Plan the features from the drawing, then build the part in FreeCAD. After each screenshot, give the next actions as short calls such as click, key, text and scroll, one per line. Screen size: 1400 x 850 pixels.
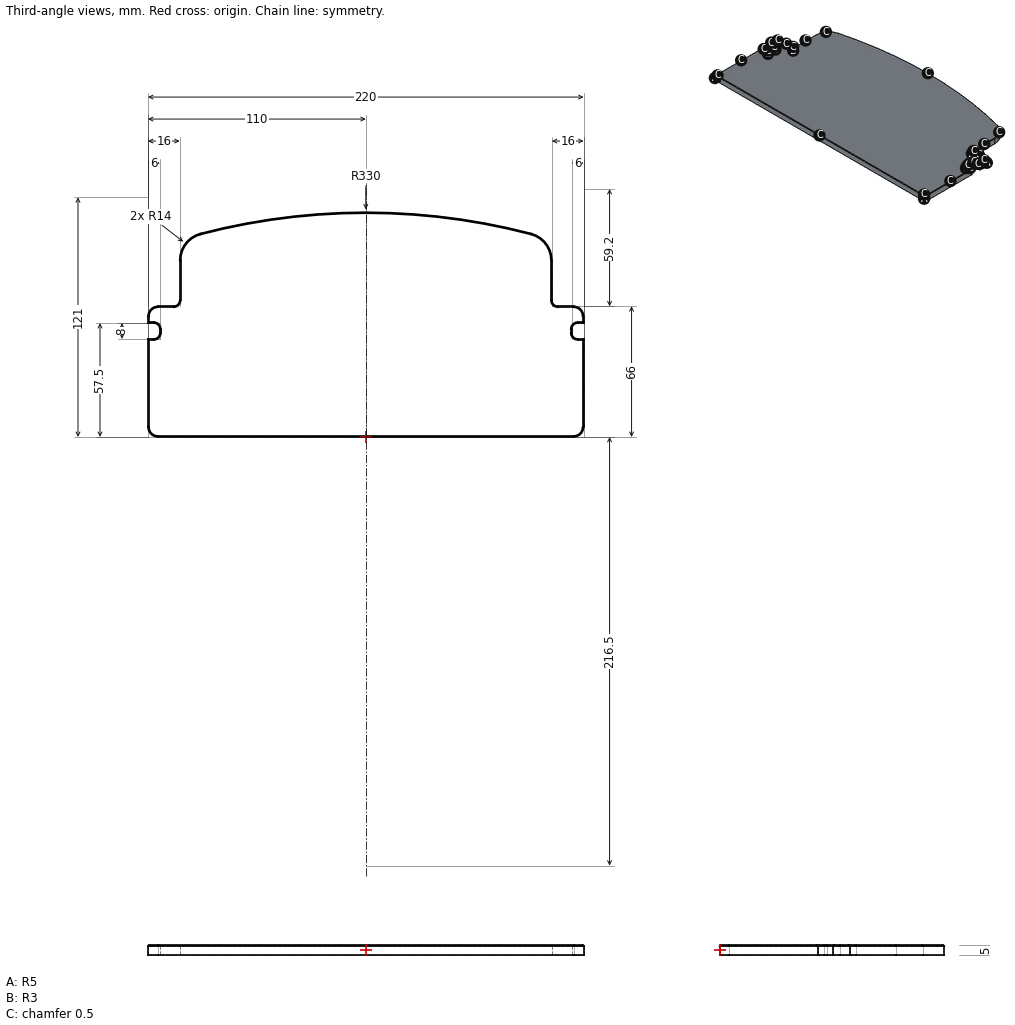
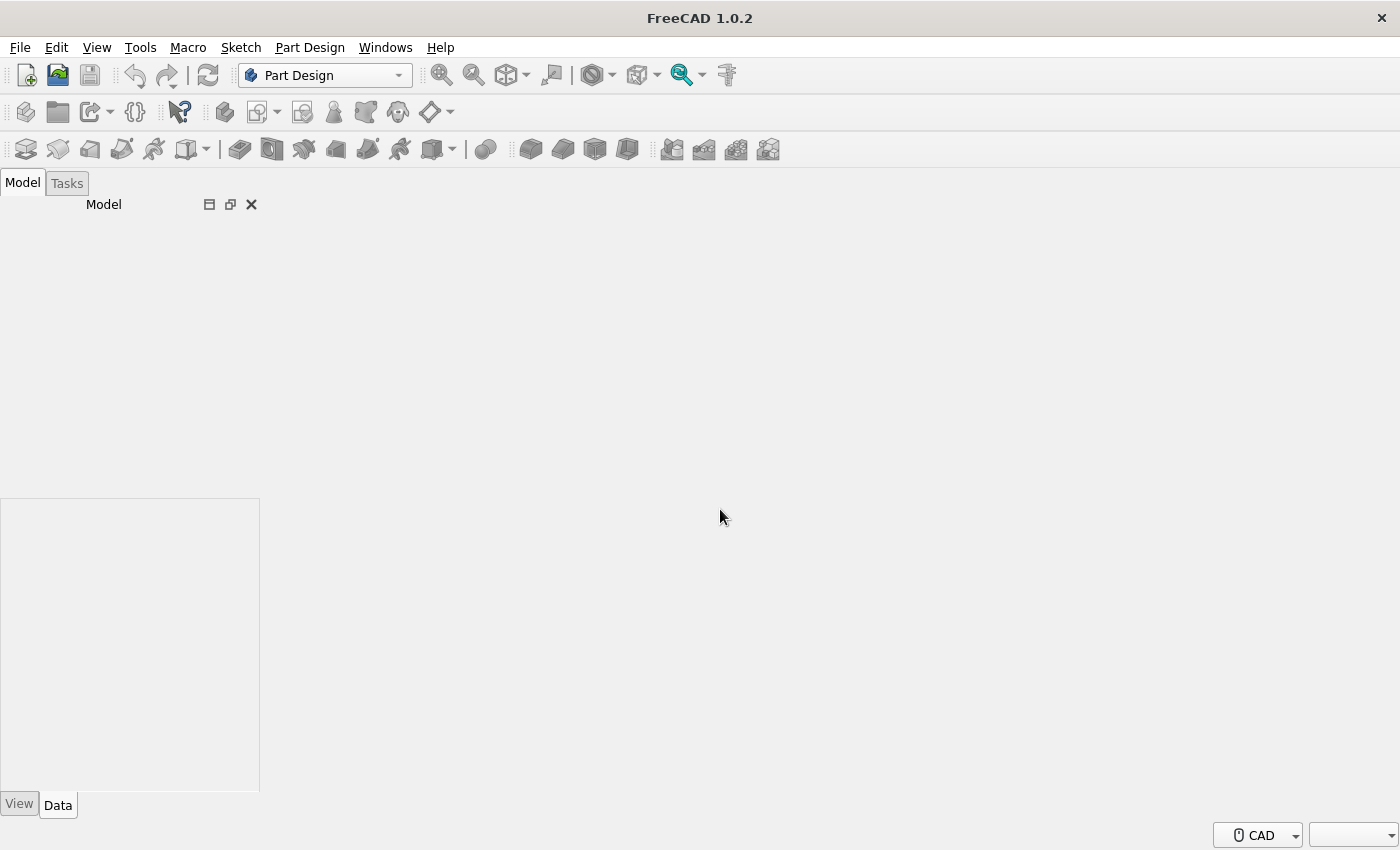
key(ctrl+n)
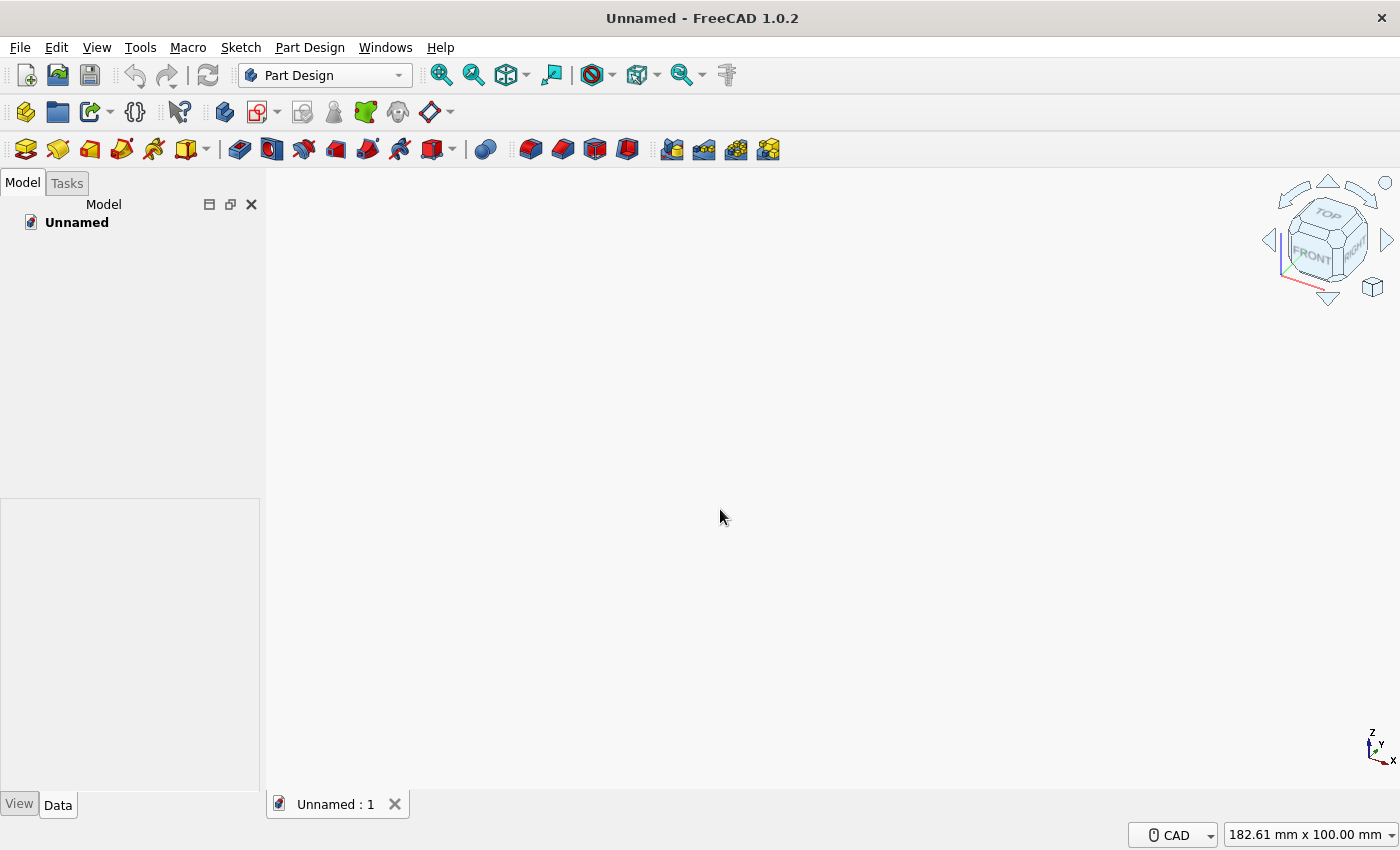
click(258, 112)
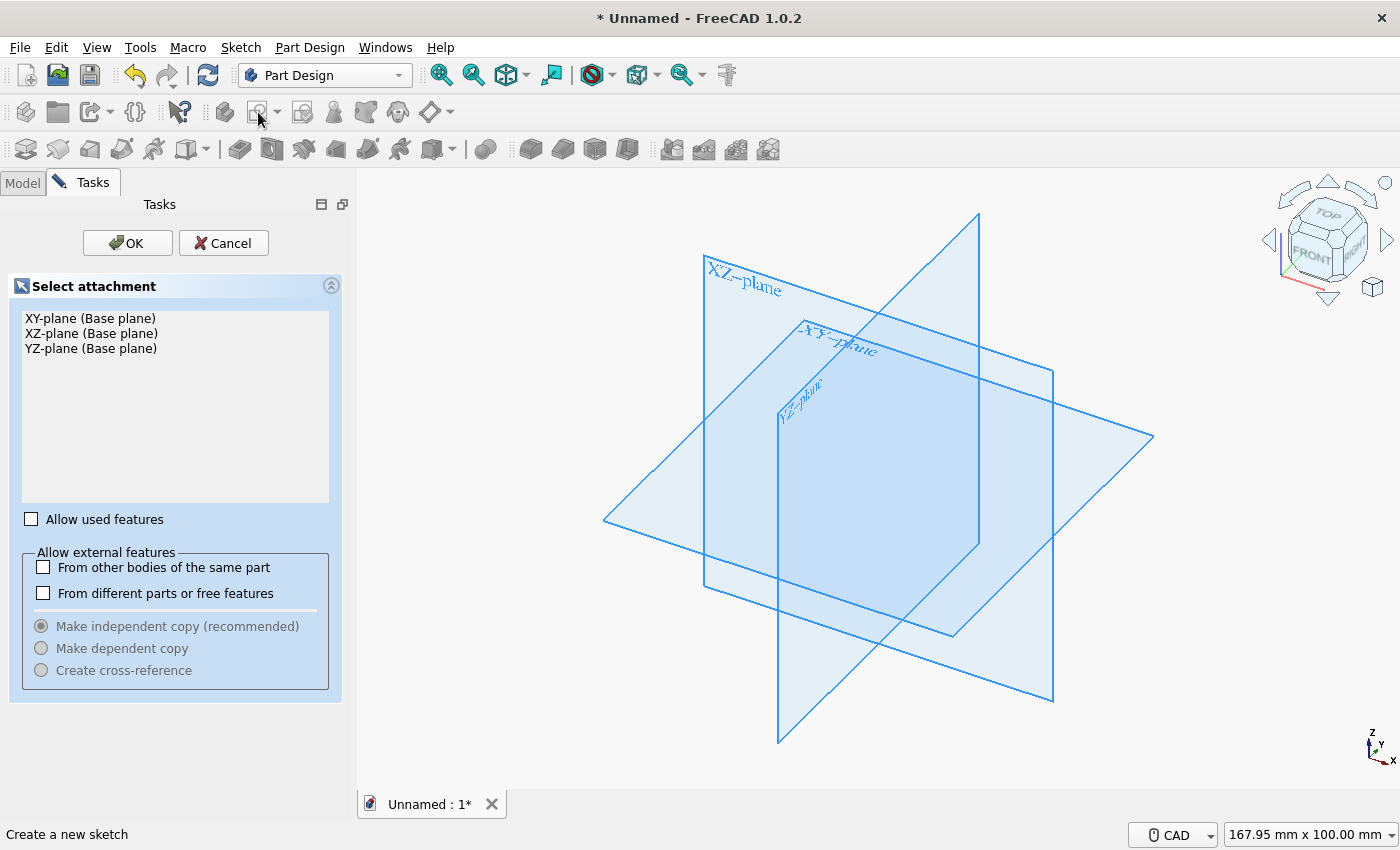
click(82, 318)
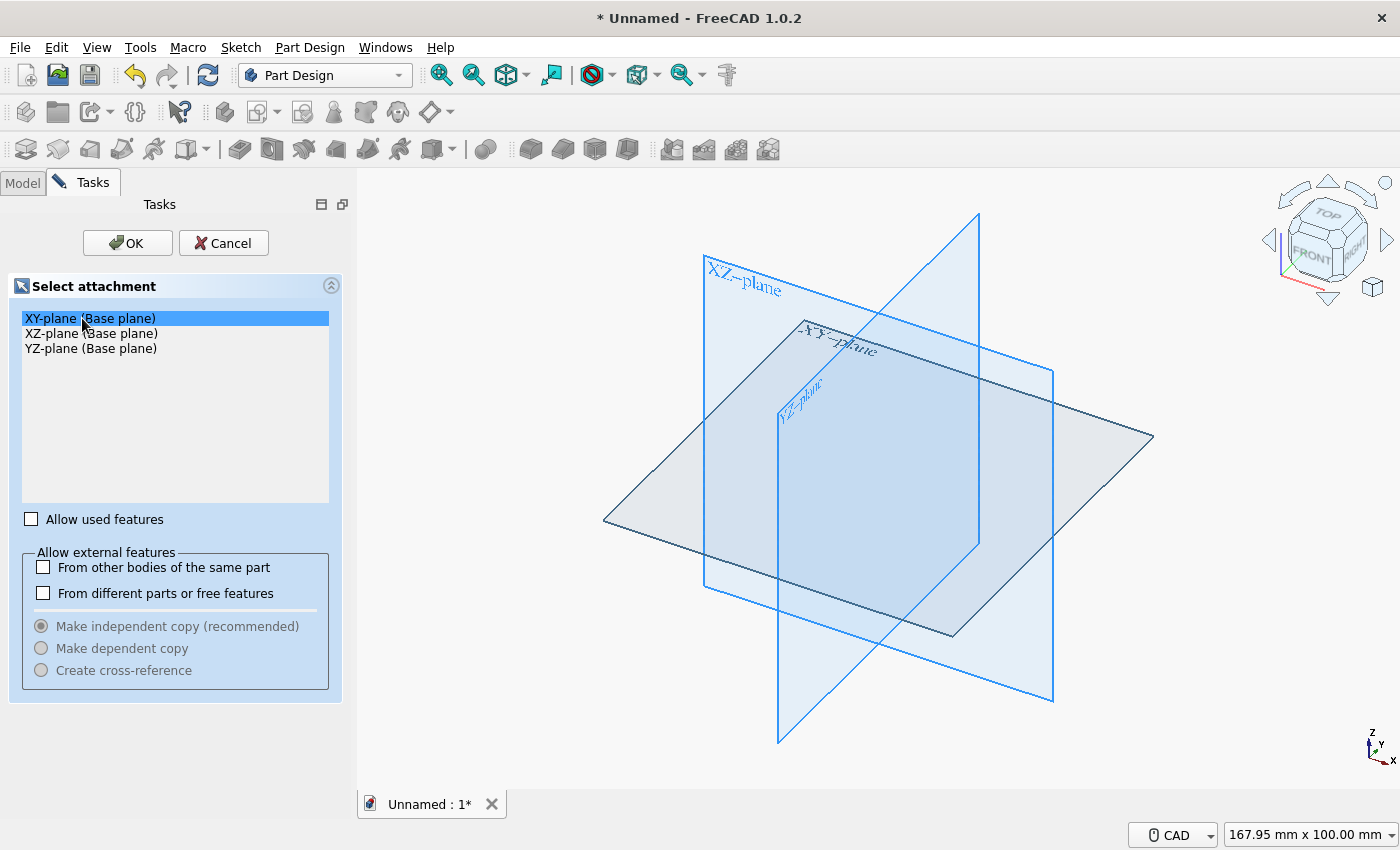
click(128, 243)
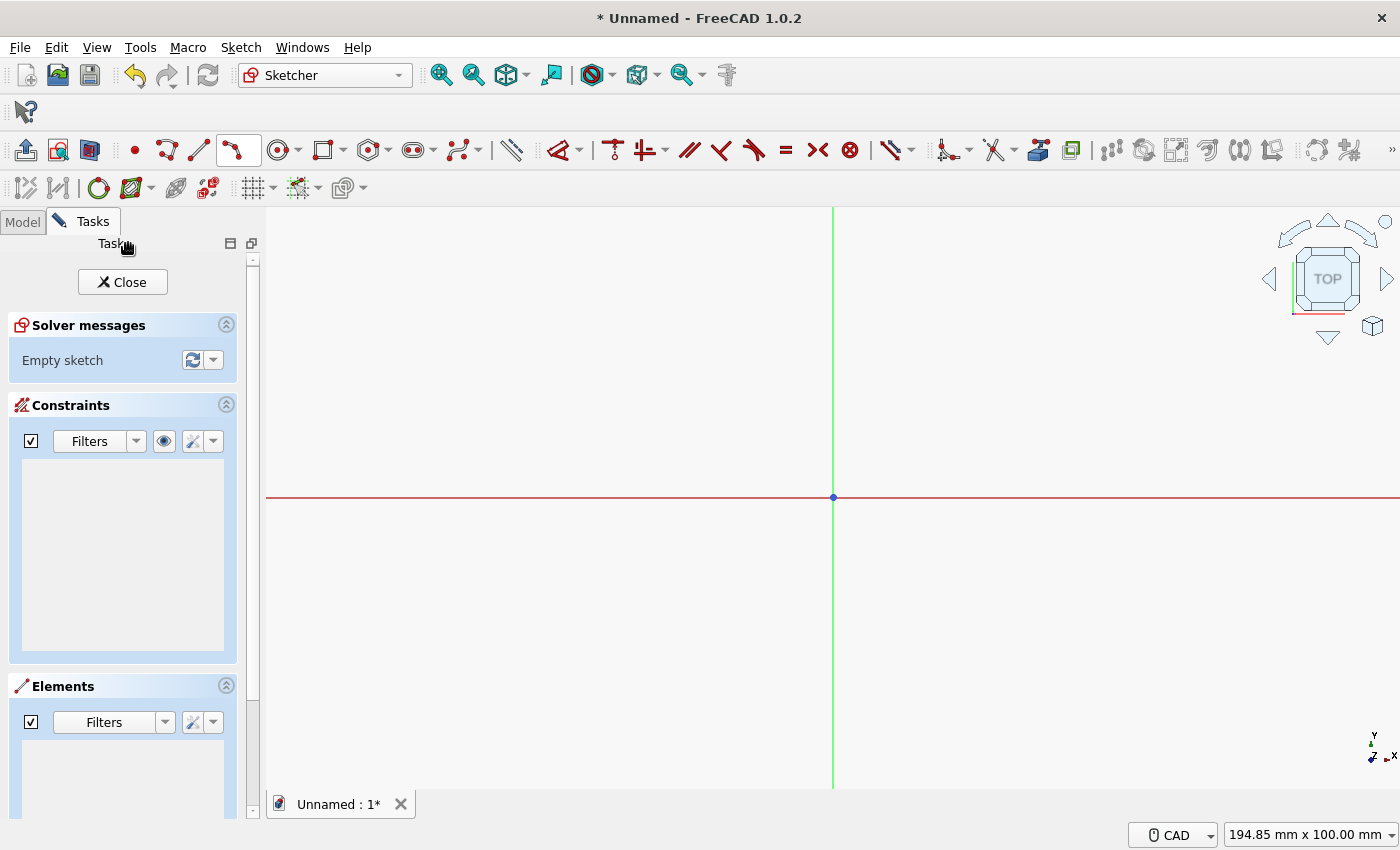
scroll(709, 761, down, 4)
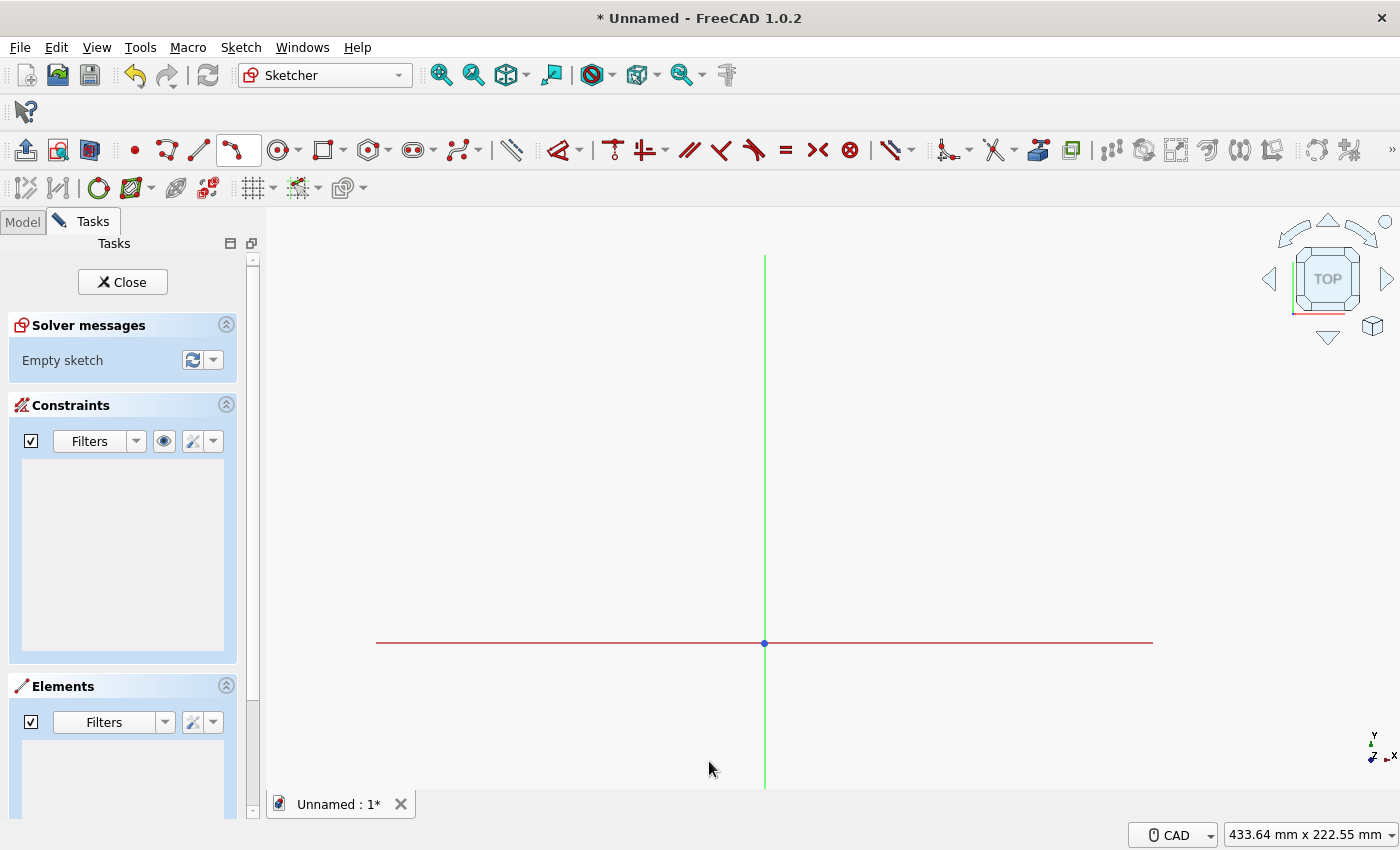
key(g)
key(r)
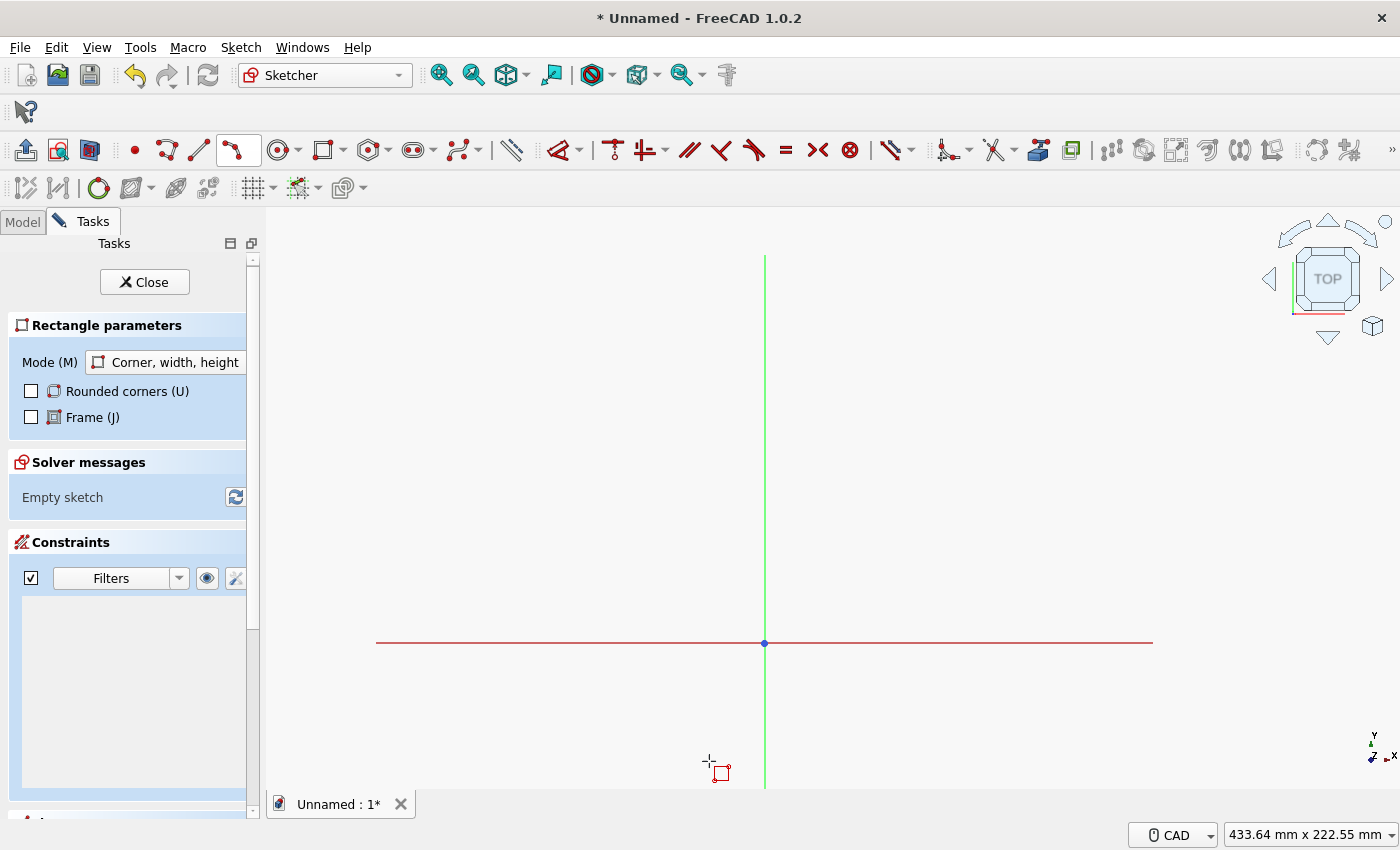
click(477, 327)
click(1053, 643)
key(Escape)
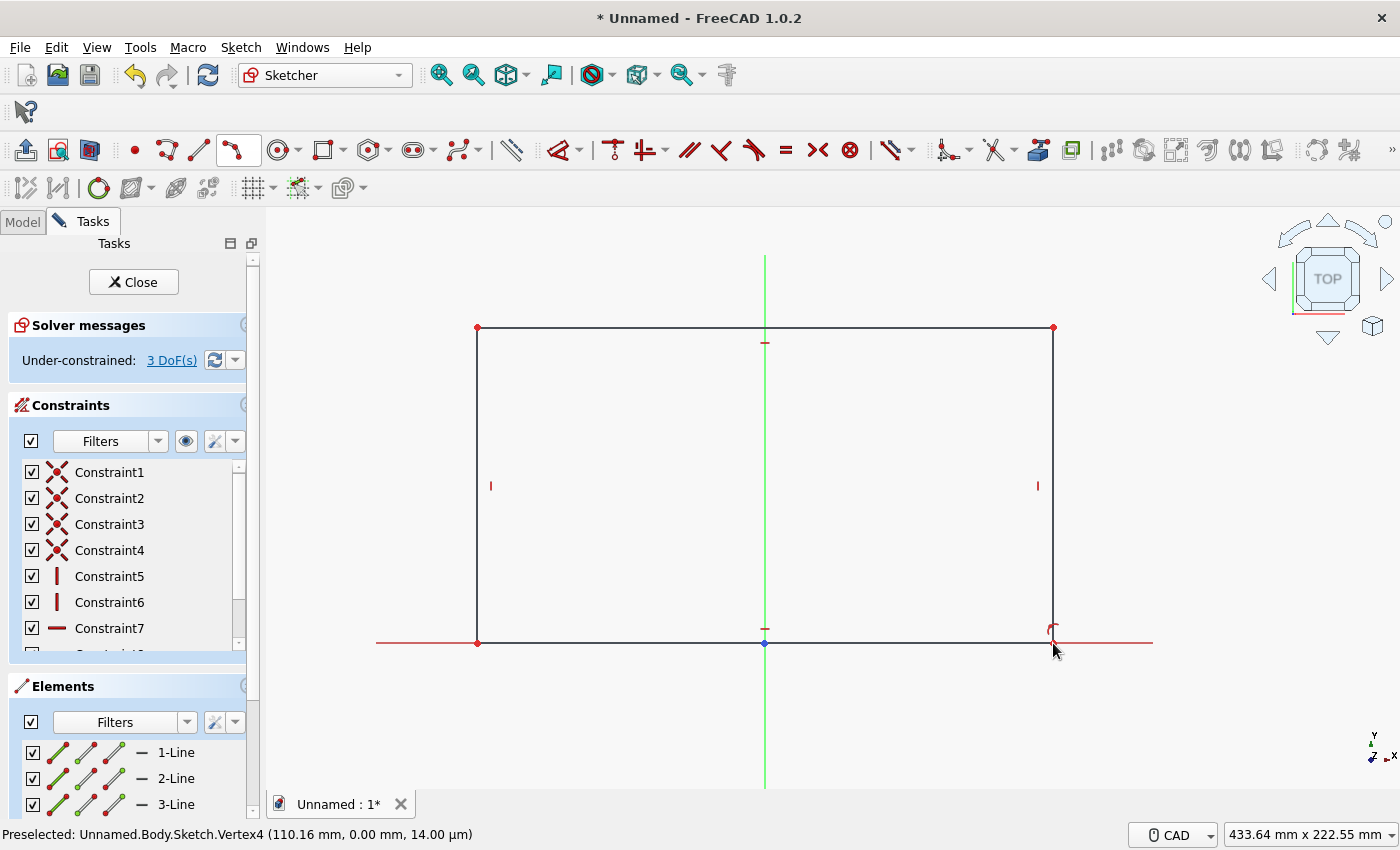
key(d)